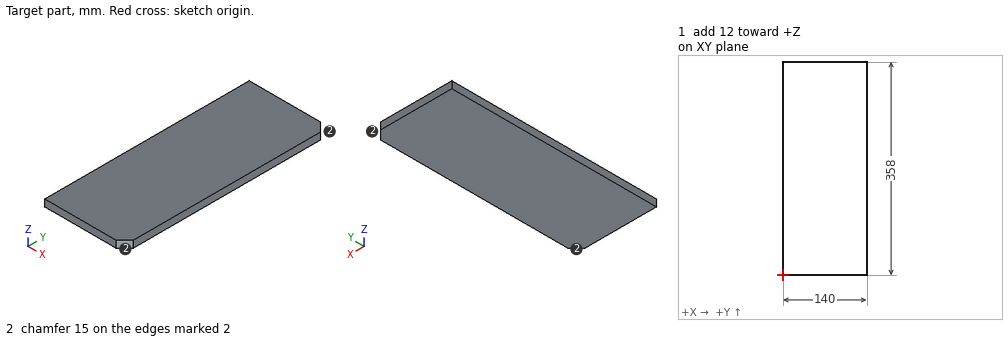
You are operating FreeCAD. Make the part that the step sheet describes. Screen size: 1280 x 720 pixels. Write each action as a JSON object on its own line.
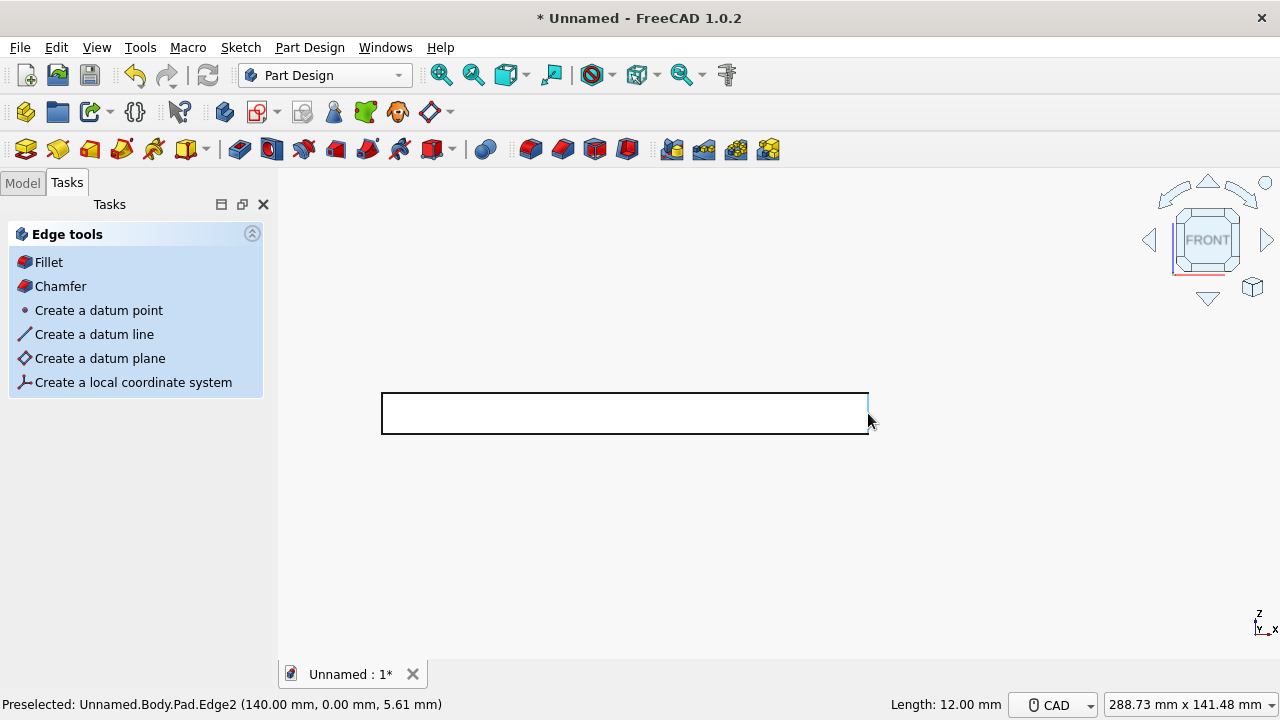
{"action": "left_click", "coordinate": [442, 76]}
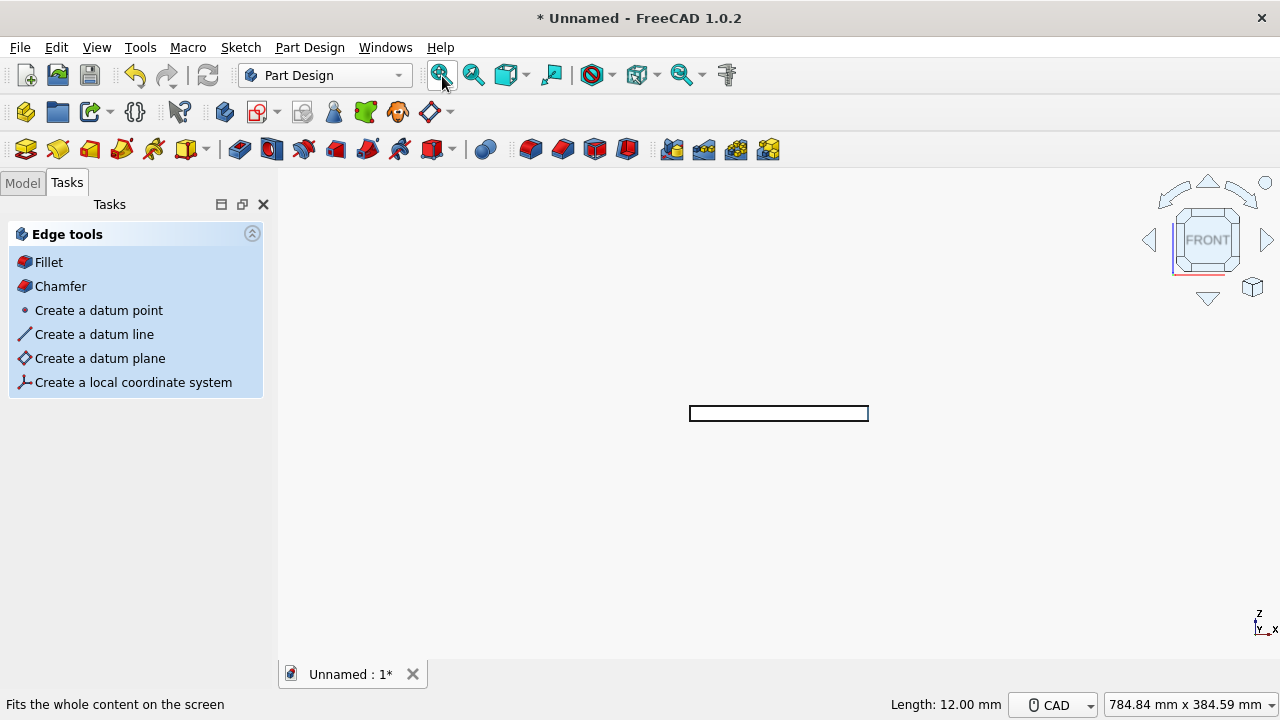
{"action": "key", "text": "3"}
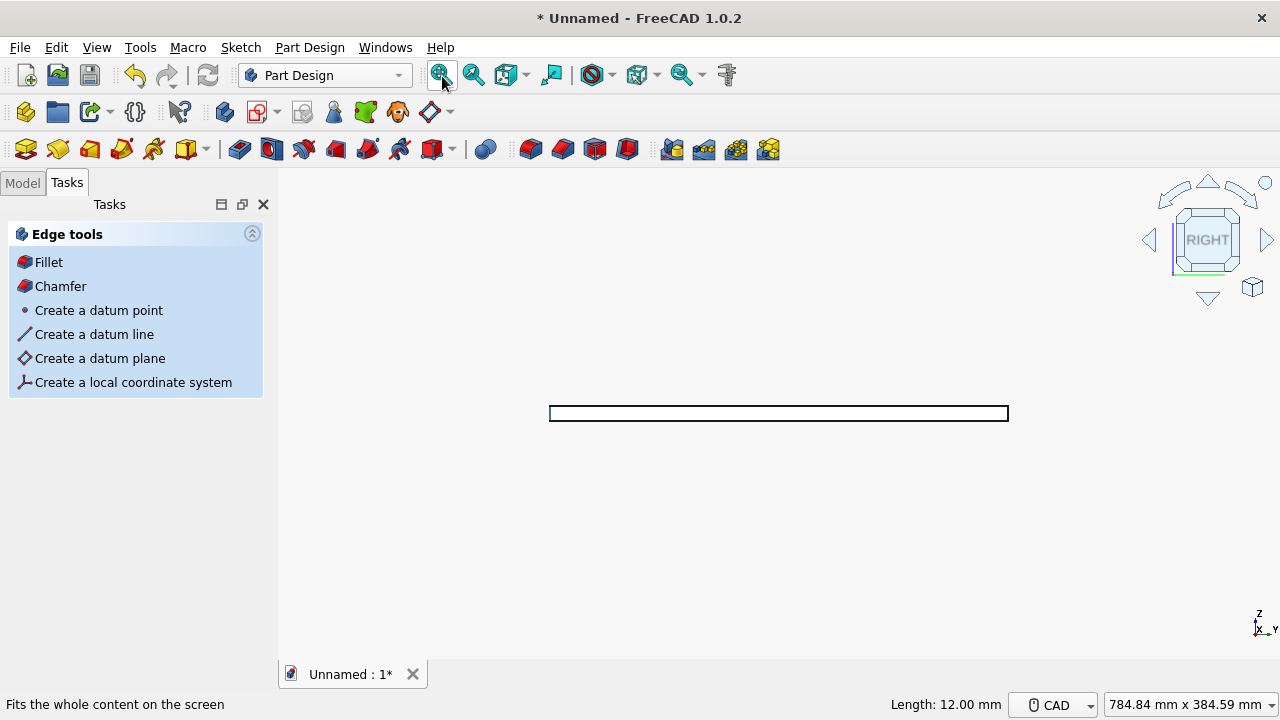
{"action": "left_click", "coordinate": [1008, 412], "text": "ctrl"}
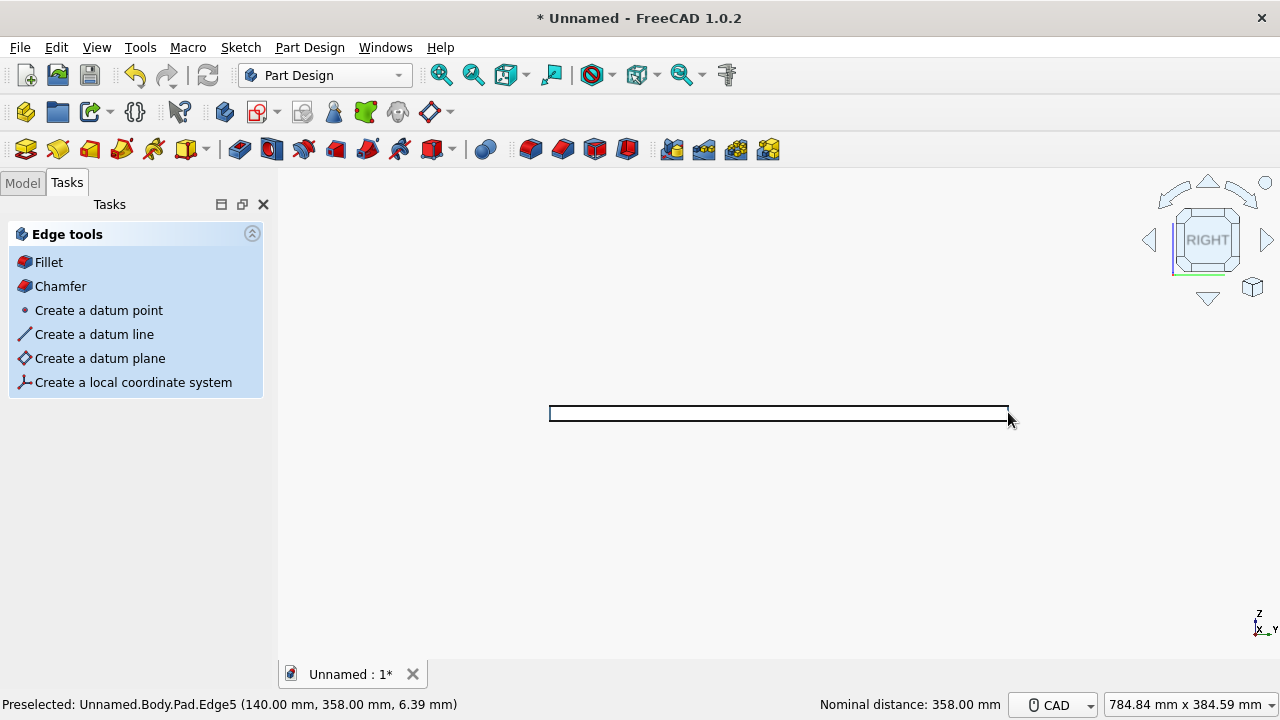
{"action": "left_click", "coordinate": [564, 150]}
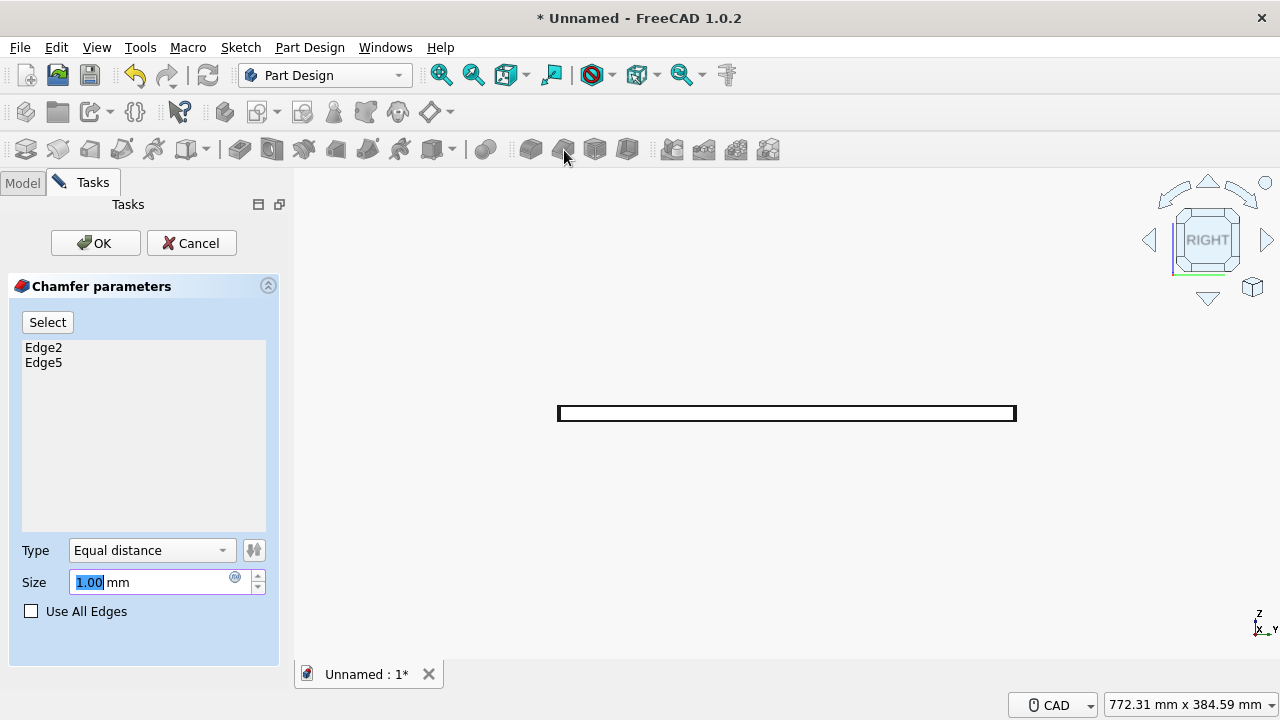
{"action": "type", "text": "15"}
{"action": "key", "text": "Tab"}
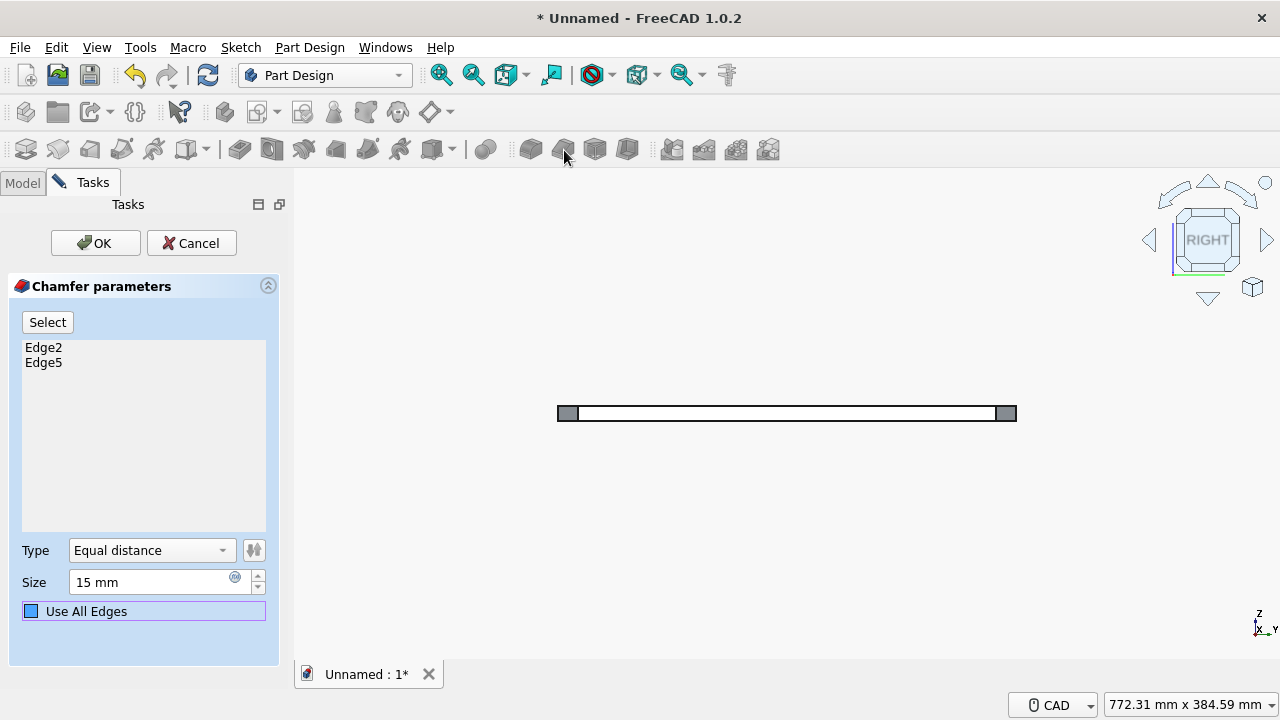
{"action": "left_click", "coordinate": [96, 243]}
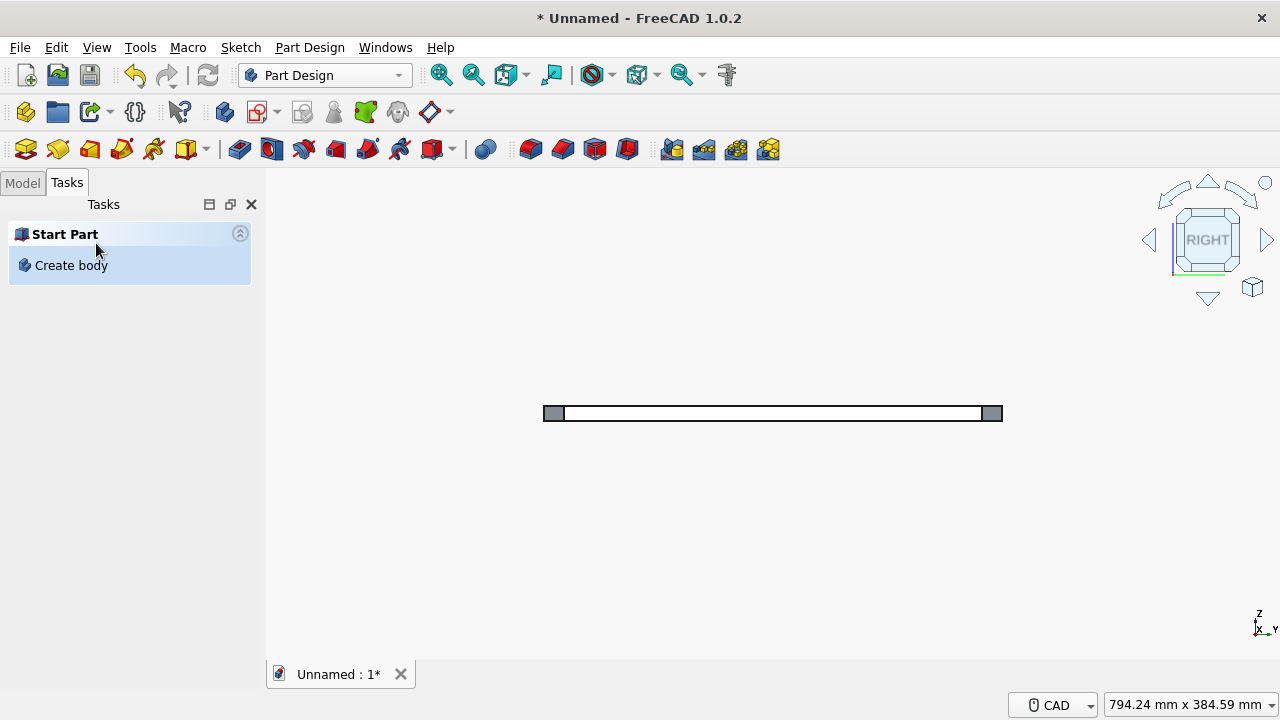
{"action": "key", "text": "0"}